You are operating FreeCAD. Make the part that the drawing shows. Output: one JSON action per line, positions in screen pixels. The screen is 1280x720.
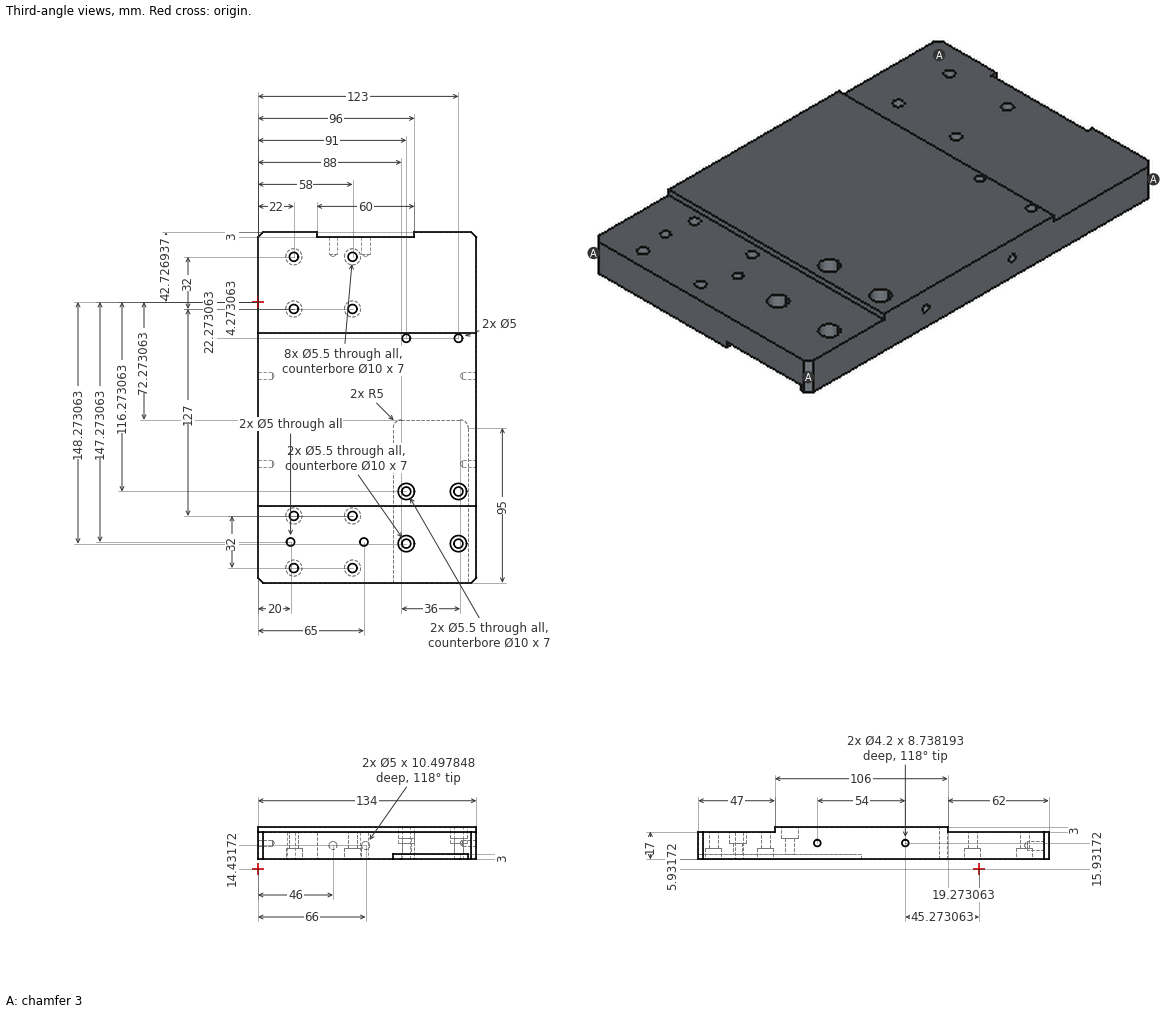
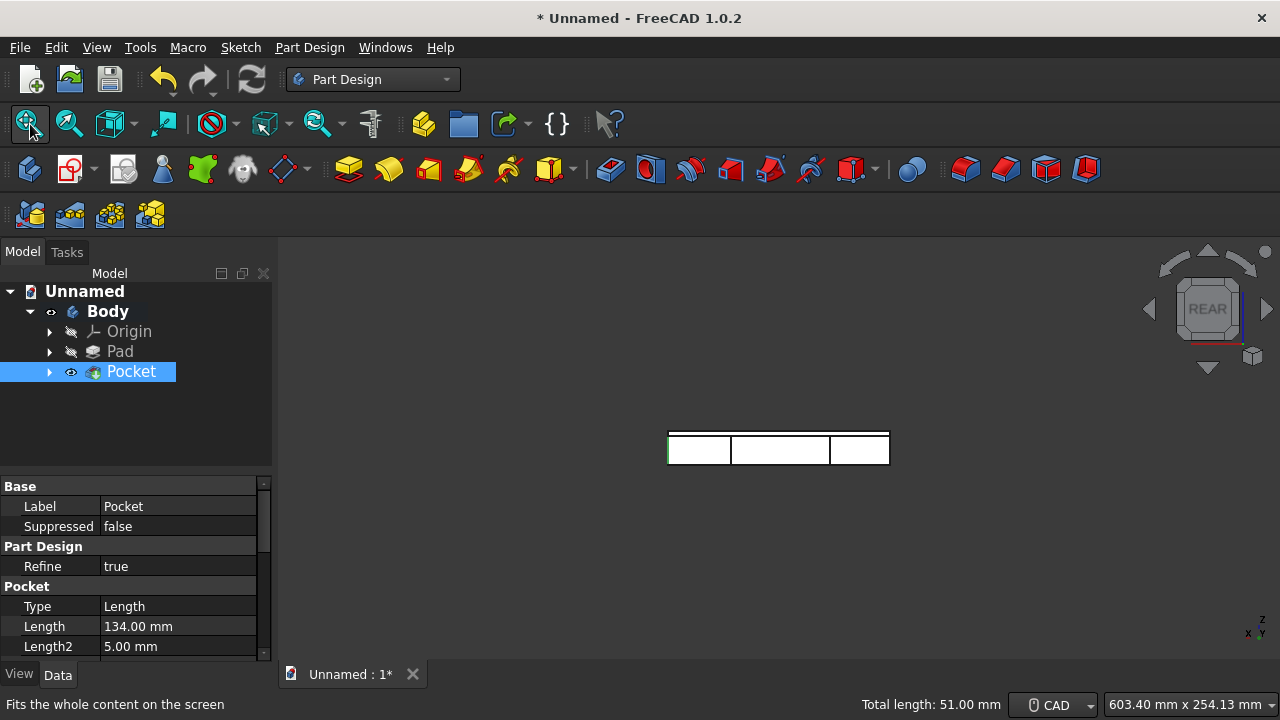
{"action": "left_click", "coordinate": [890, 449], "text": "ctrl"}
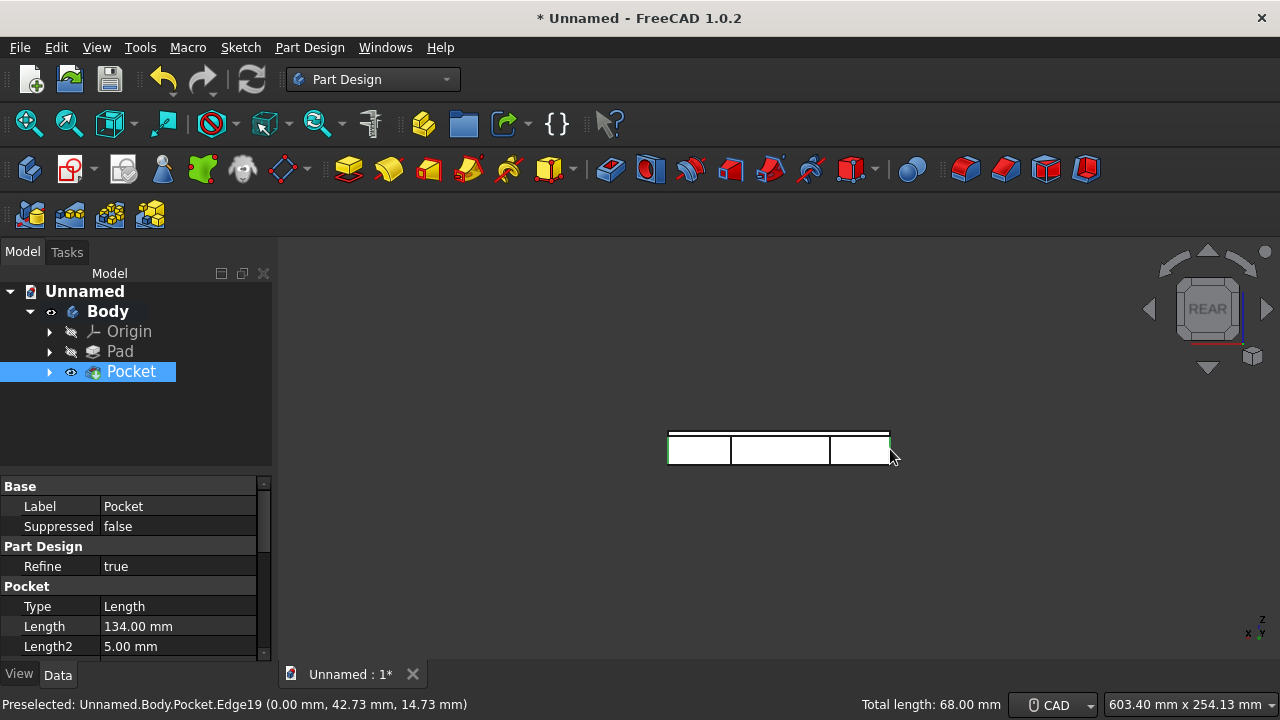
{"action": "left_click", "coordinate": [1006, 170]}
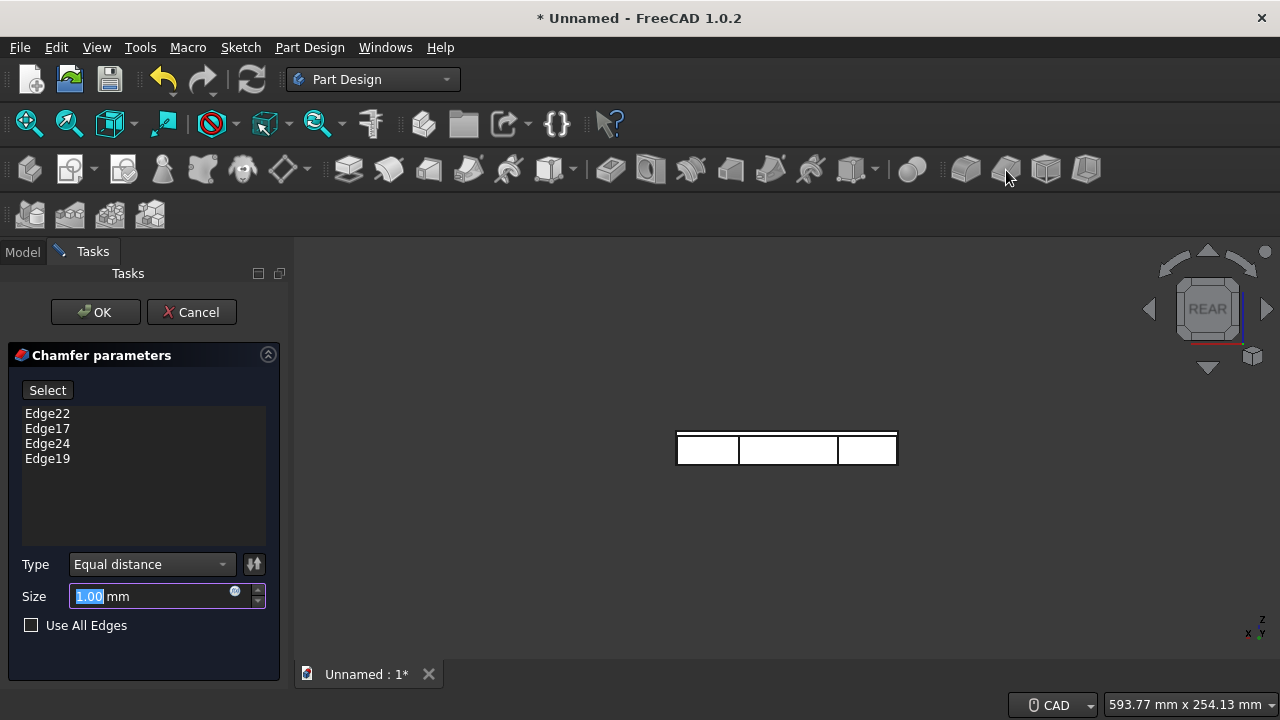
{"action": "type", "text": "3"}
{"action": "key", "text": "Tab"}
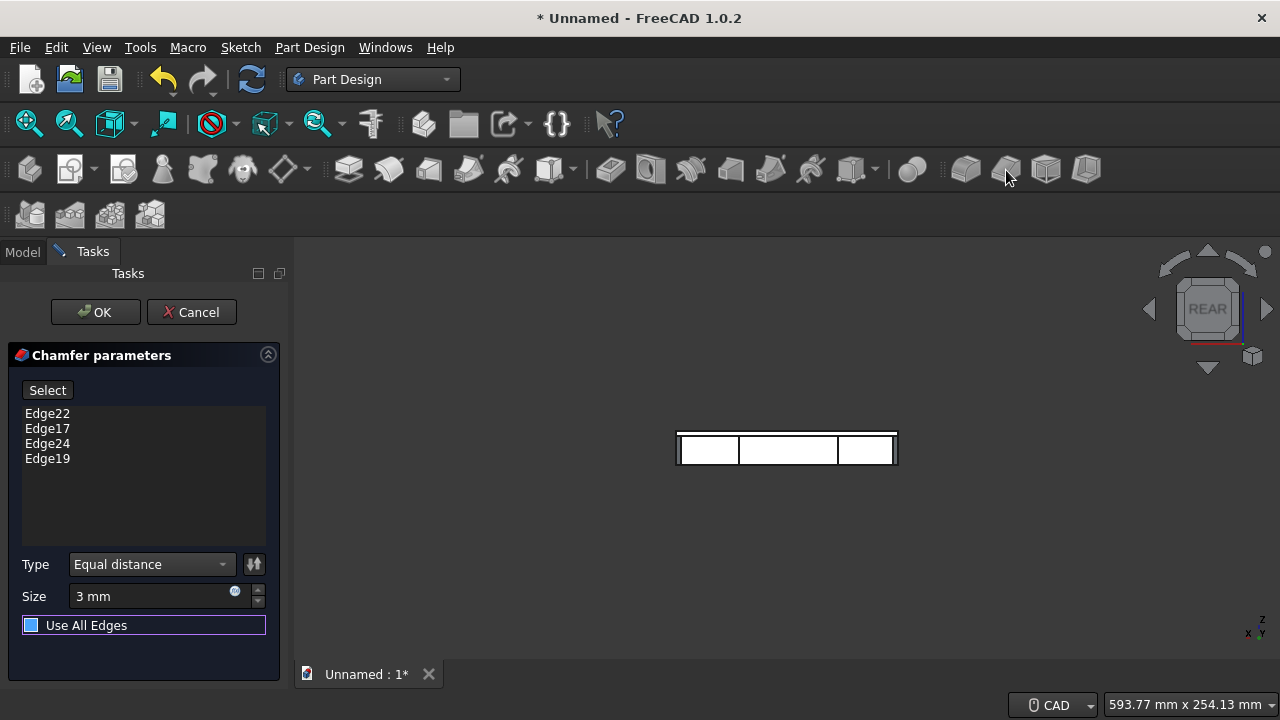
{"action": "left_click", "coordinate": [96, 312]}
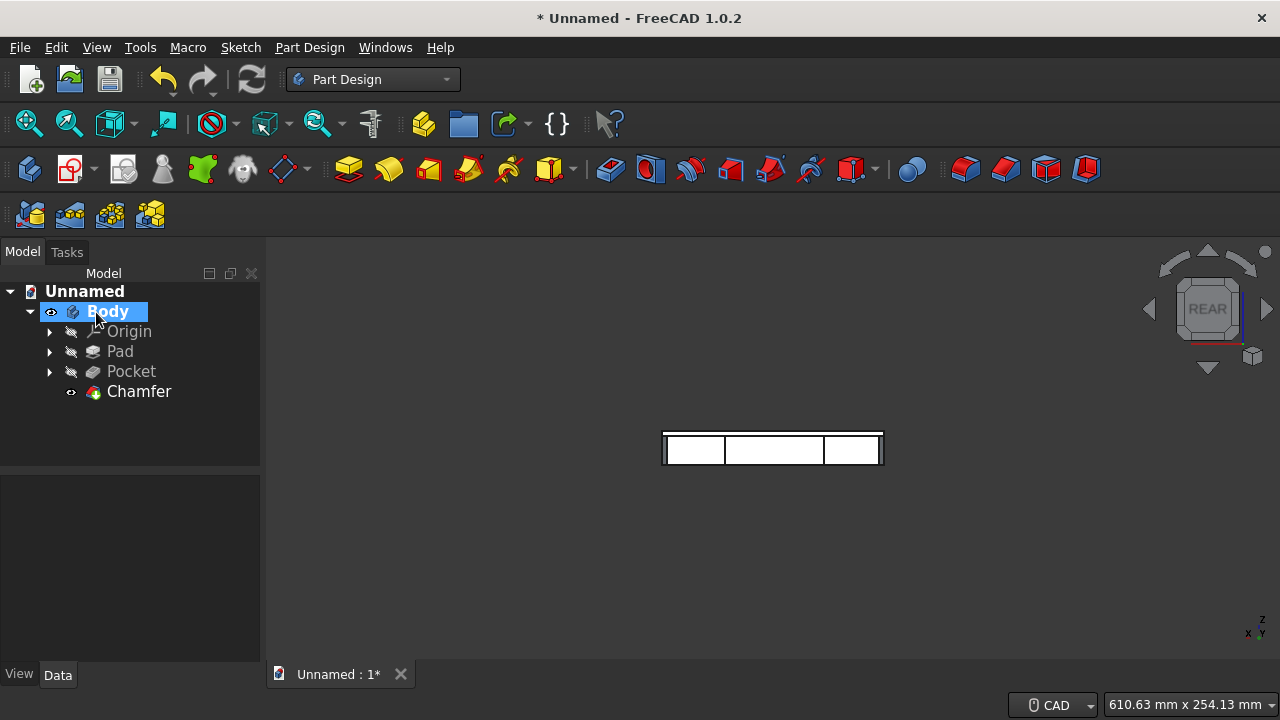
{"action": "left_click", "coordinate": [30, 124]}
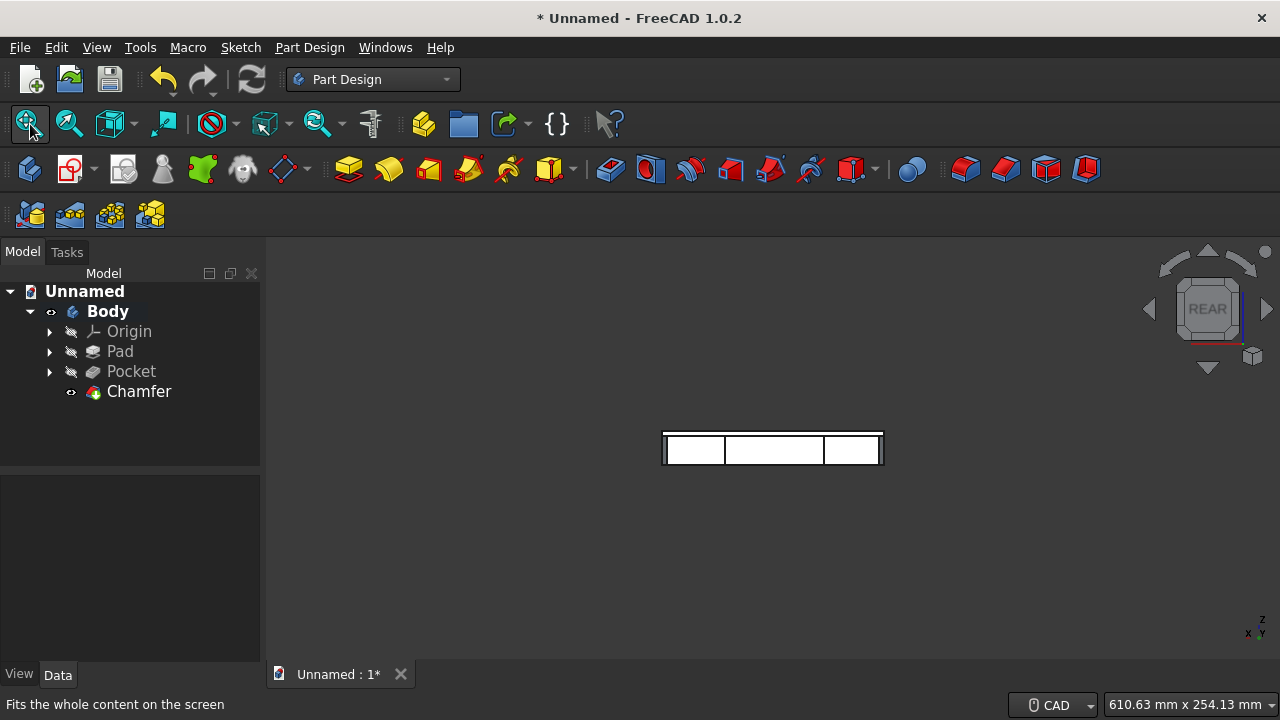
{"action": "key", "text": "0"}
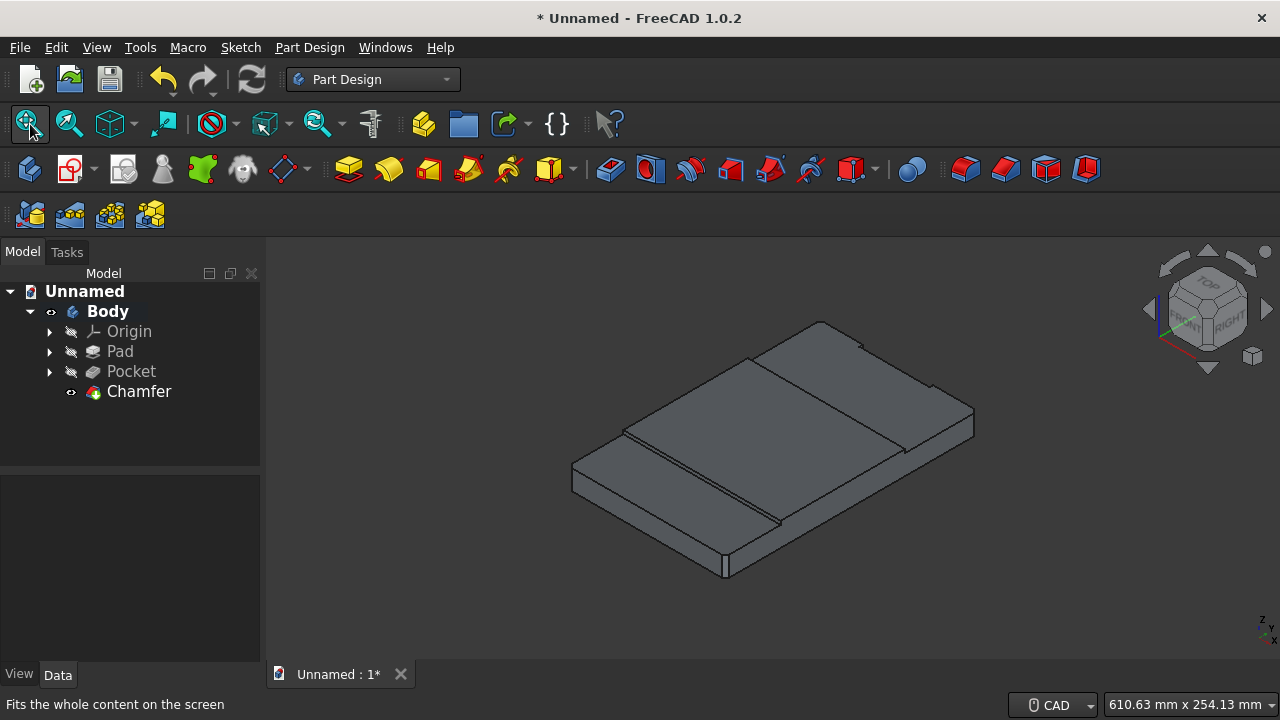
{"action": "left_click", "coordinate": [887, 472]}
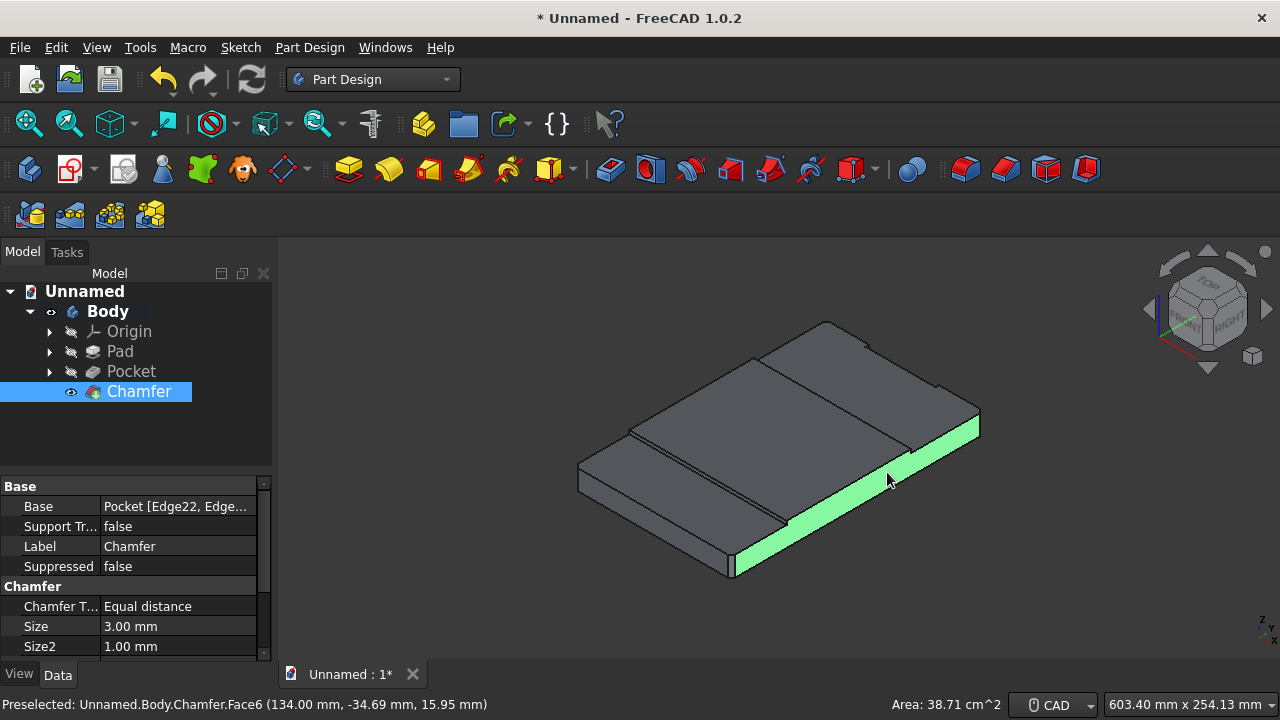
{"action": "left_click", "coordinate": [70, 170]}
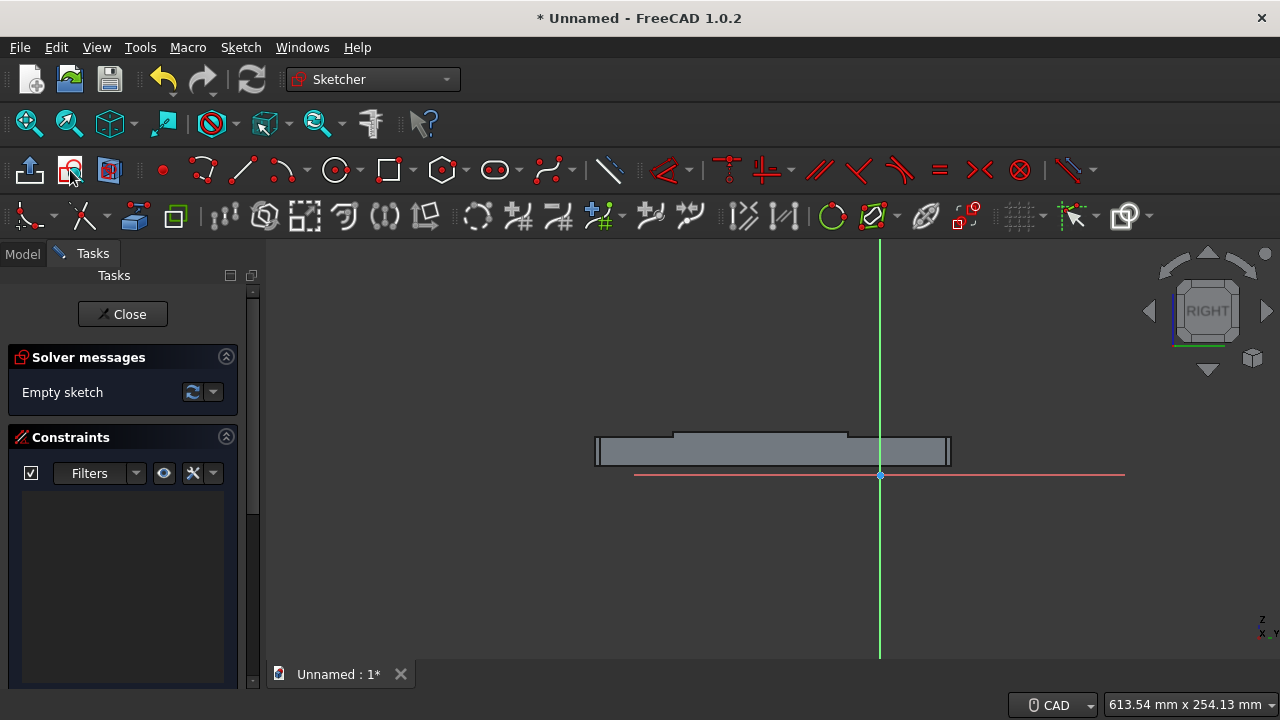
{"action": "scroll", "coordinate": [836, 465], "scroll_direction": "up", "scroll_amount": 6}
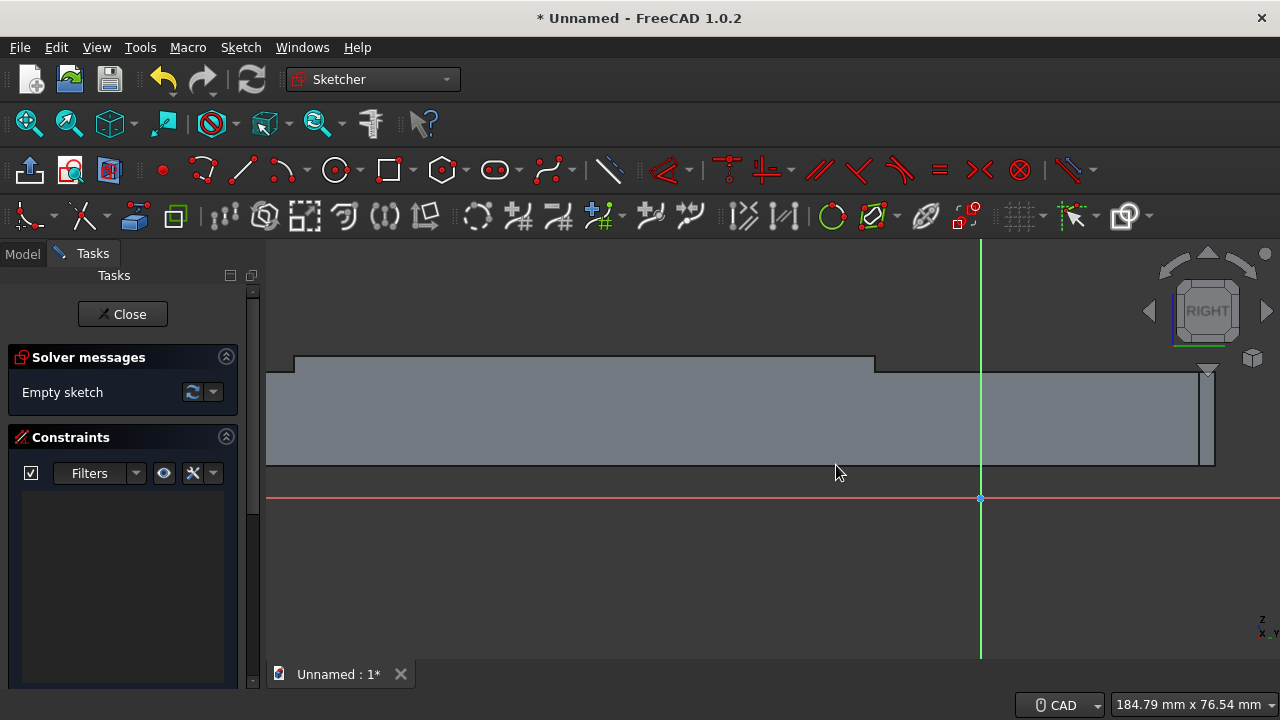
{"action": "left_click", "coordinate": [336, 170]}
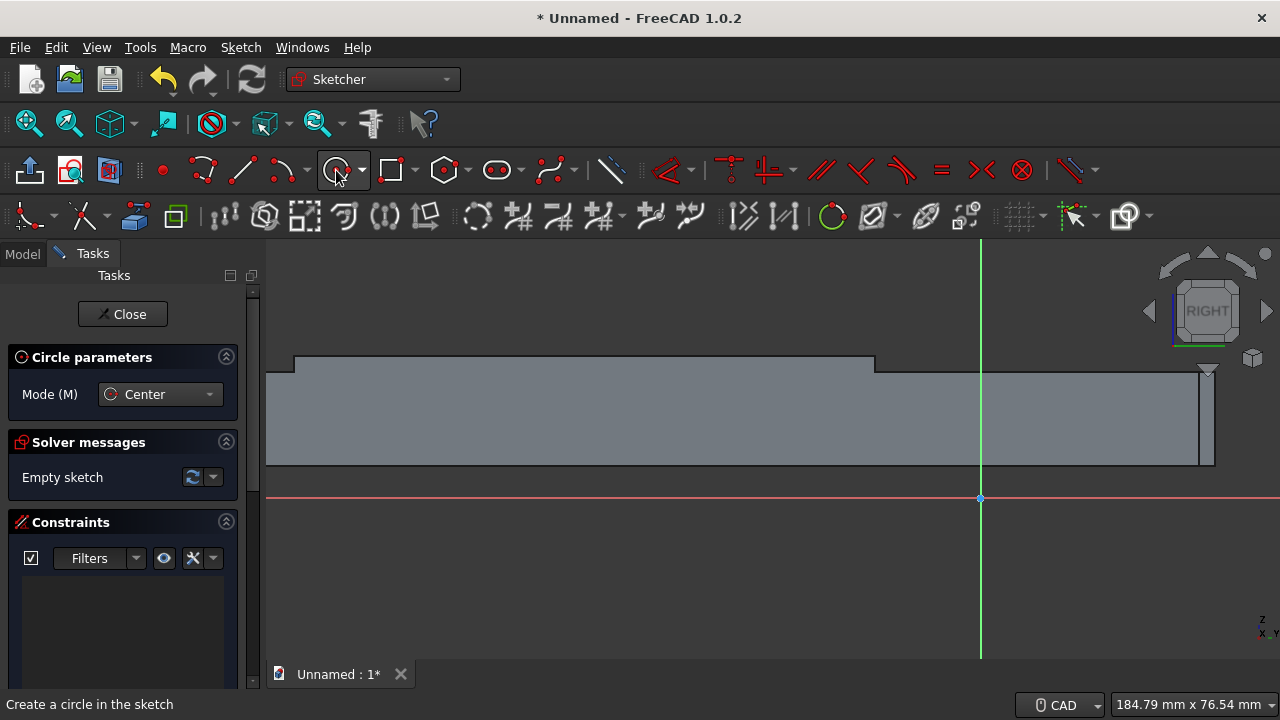
{"action": "scroll", "coordinate": [733, 411], "scroll_direction": "up", "scroll_amount": 4}